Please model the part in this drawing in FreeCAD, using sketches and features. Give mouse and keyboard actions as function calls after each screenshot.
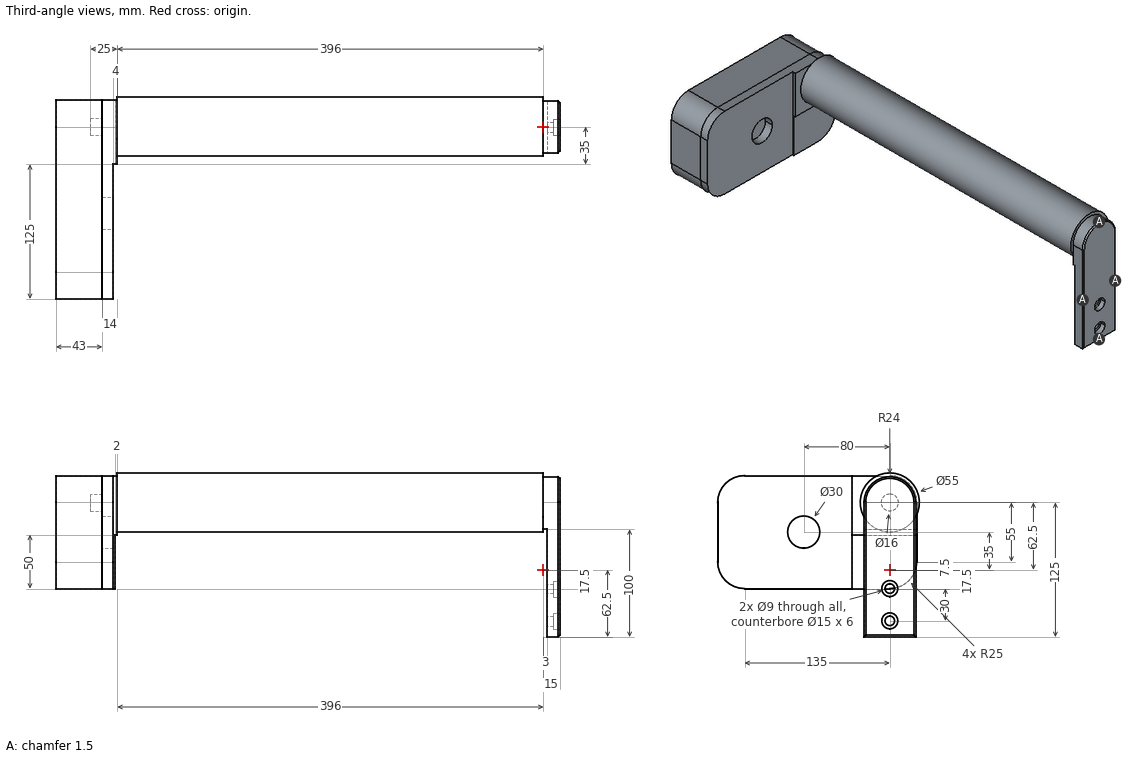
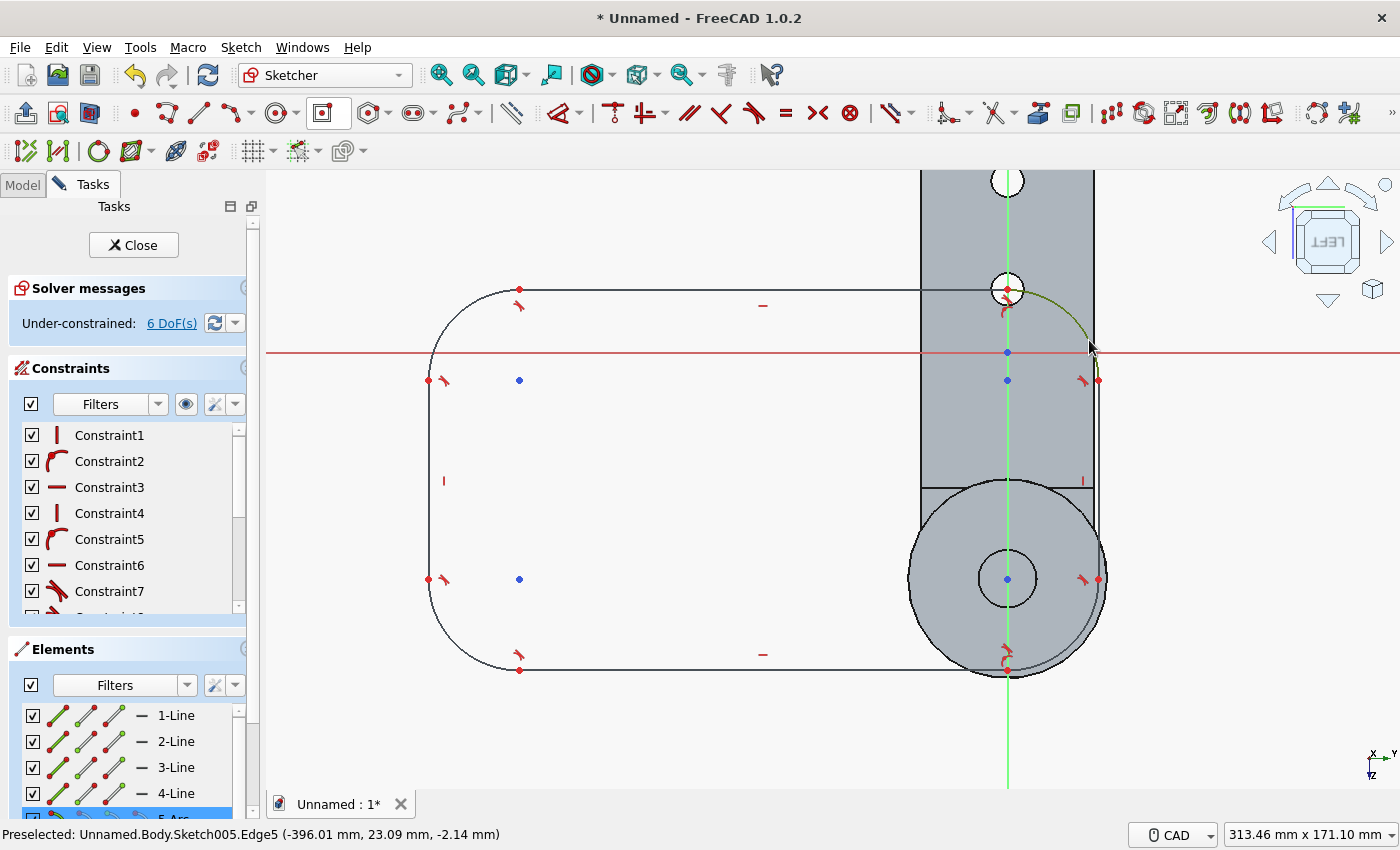
click(479, 300)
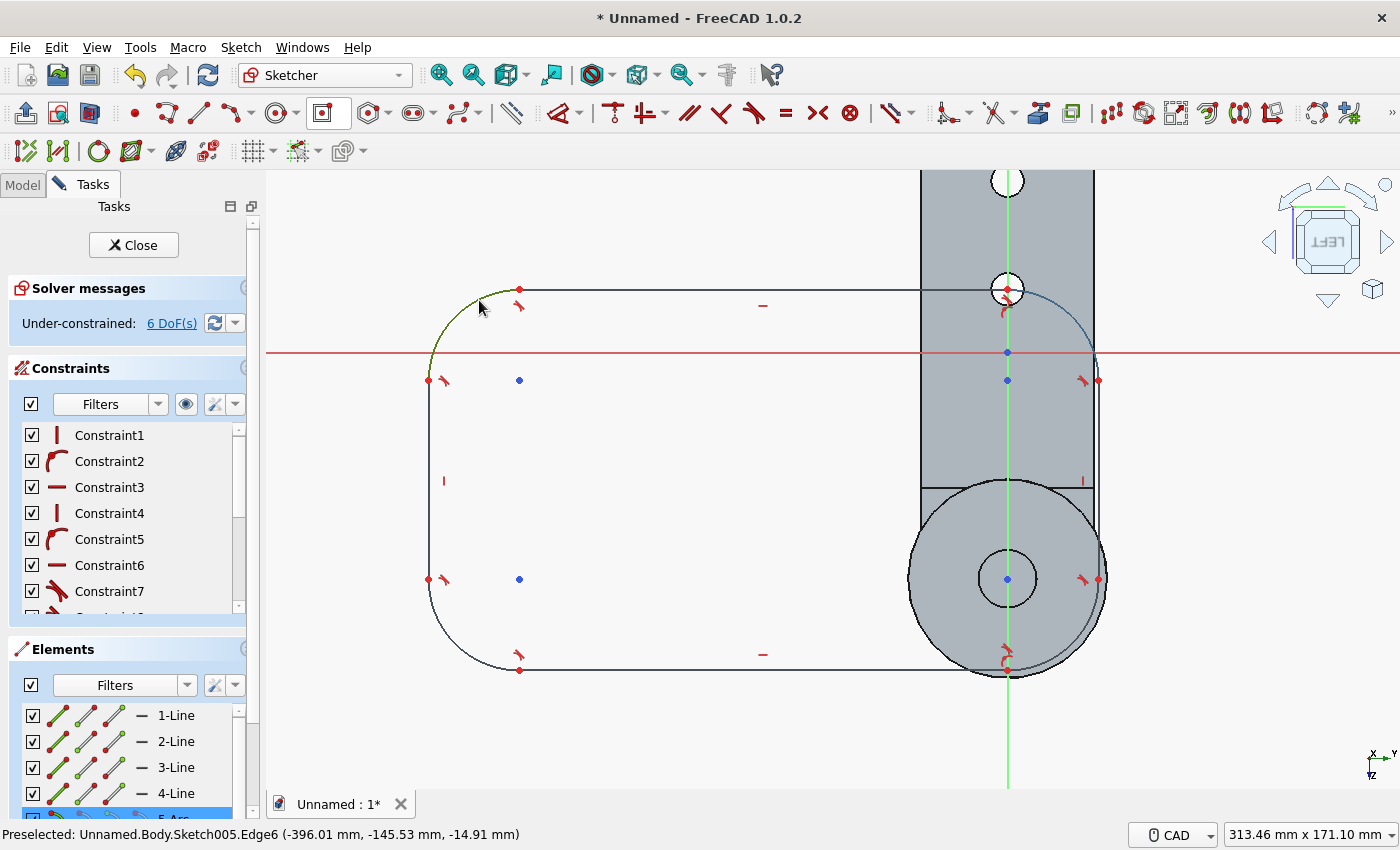
click(439, 621)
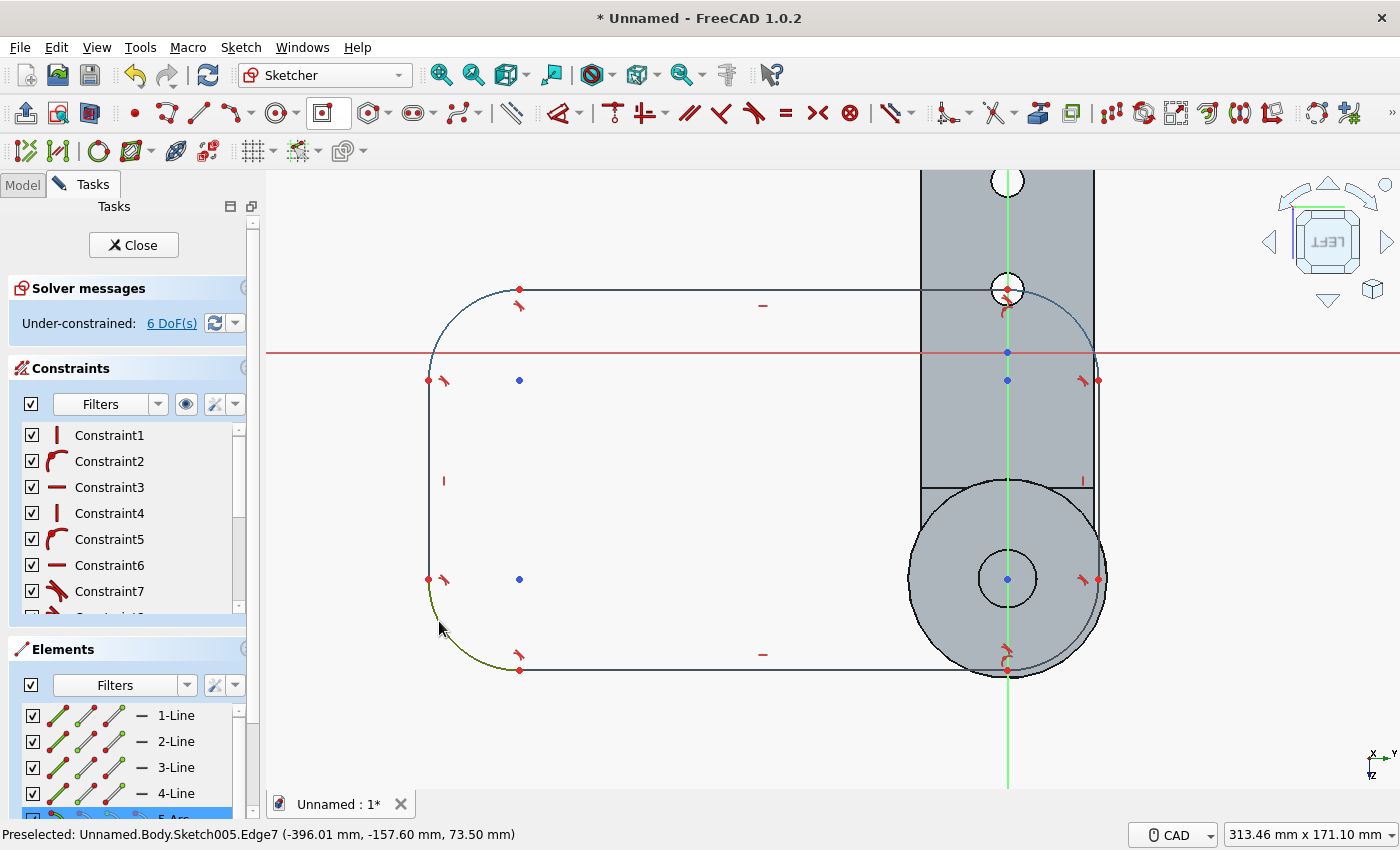
key(e)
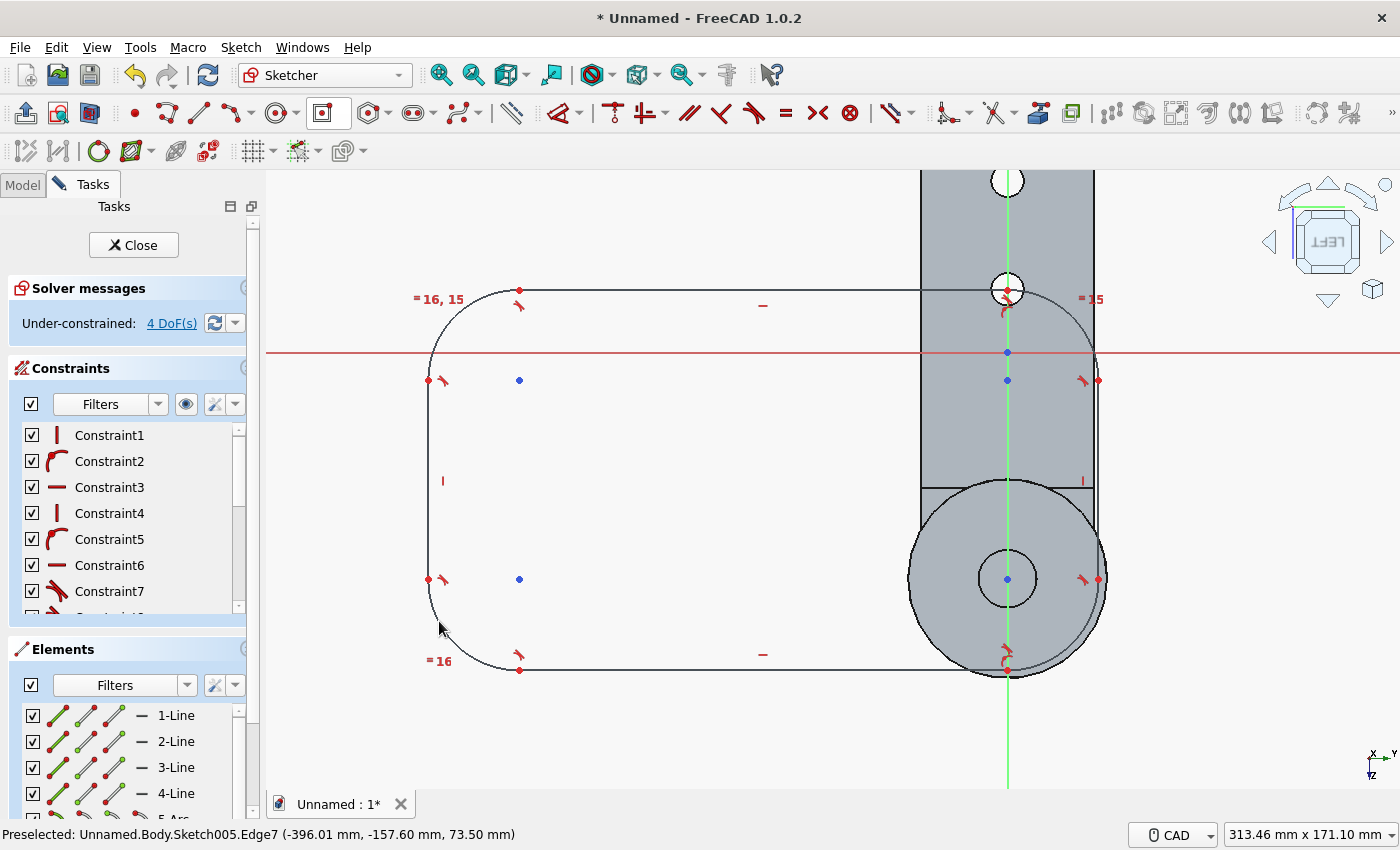
click(558, 114)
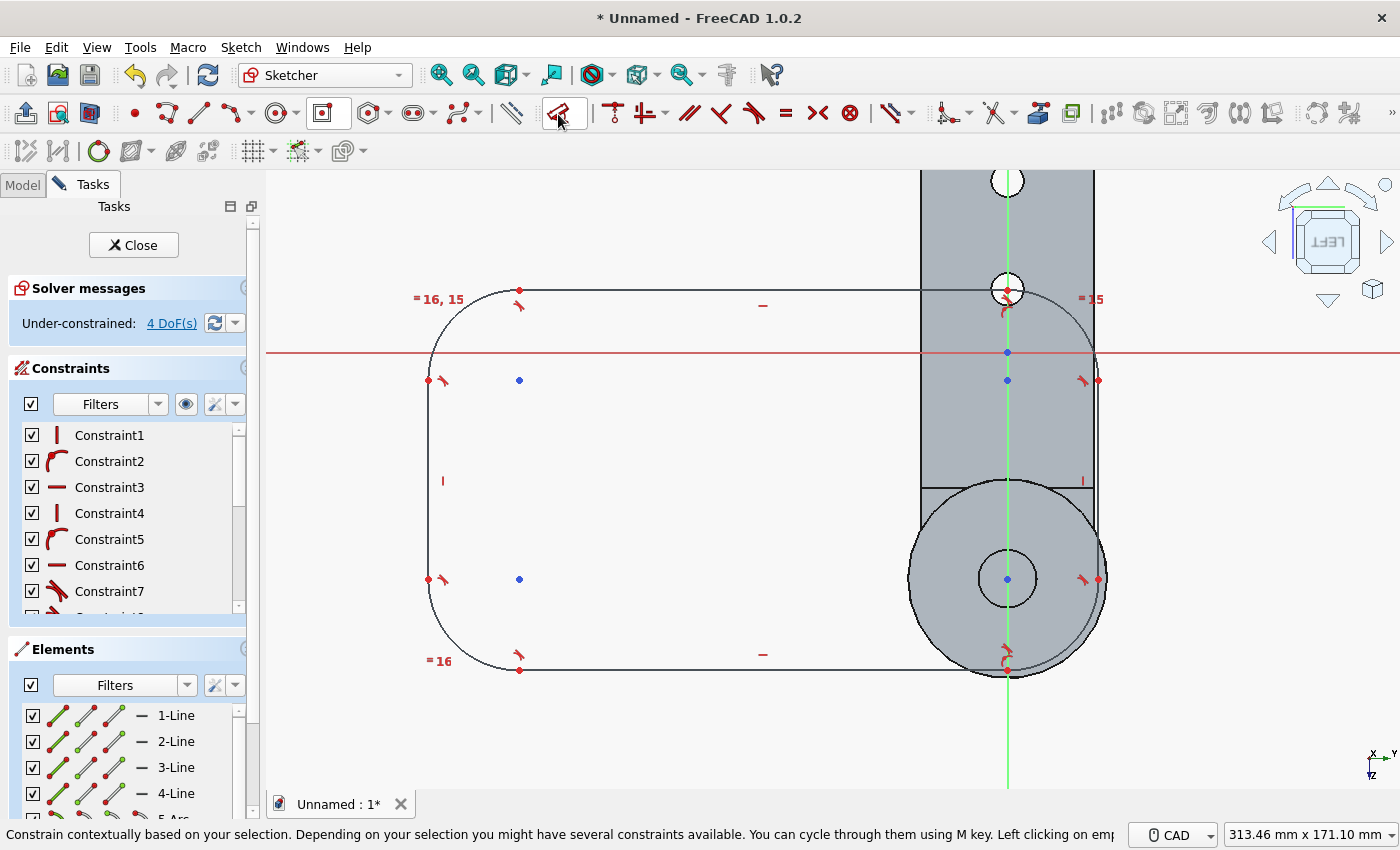
click(1089, 340)
click(1118, 326)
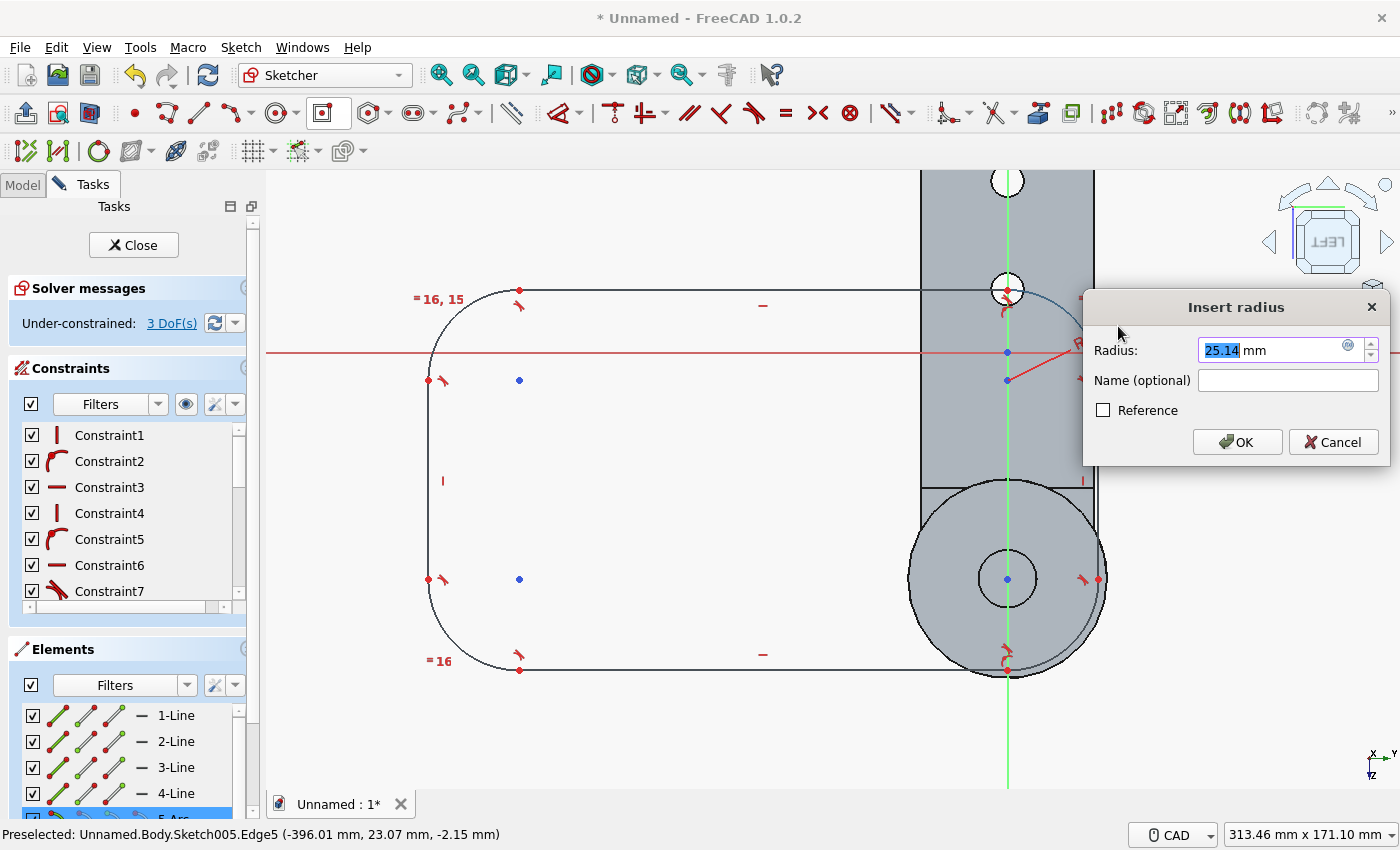
text(25)
key(Return)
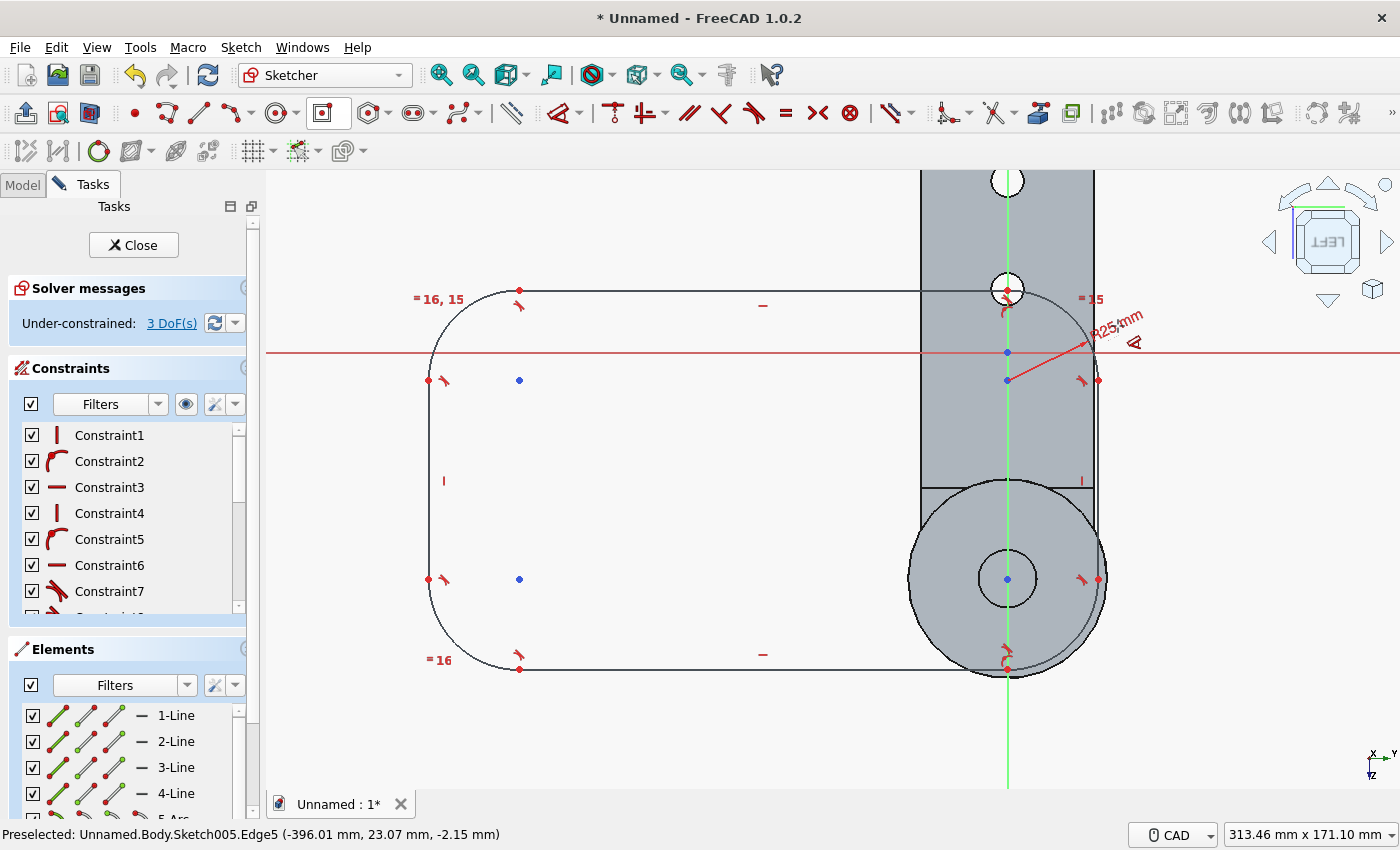
click(1098, 520)
click(1132, 480)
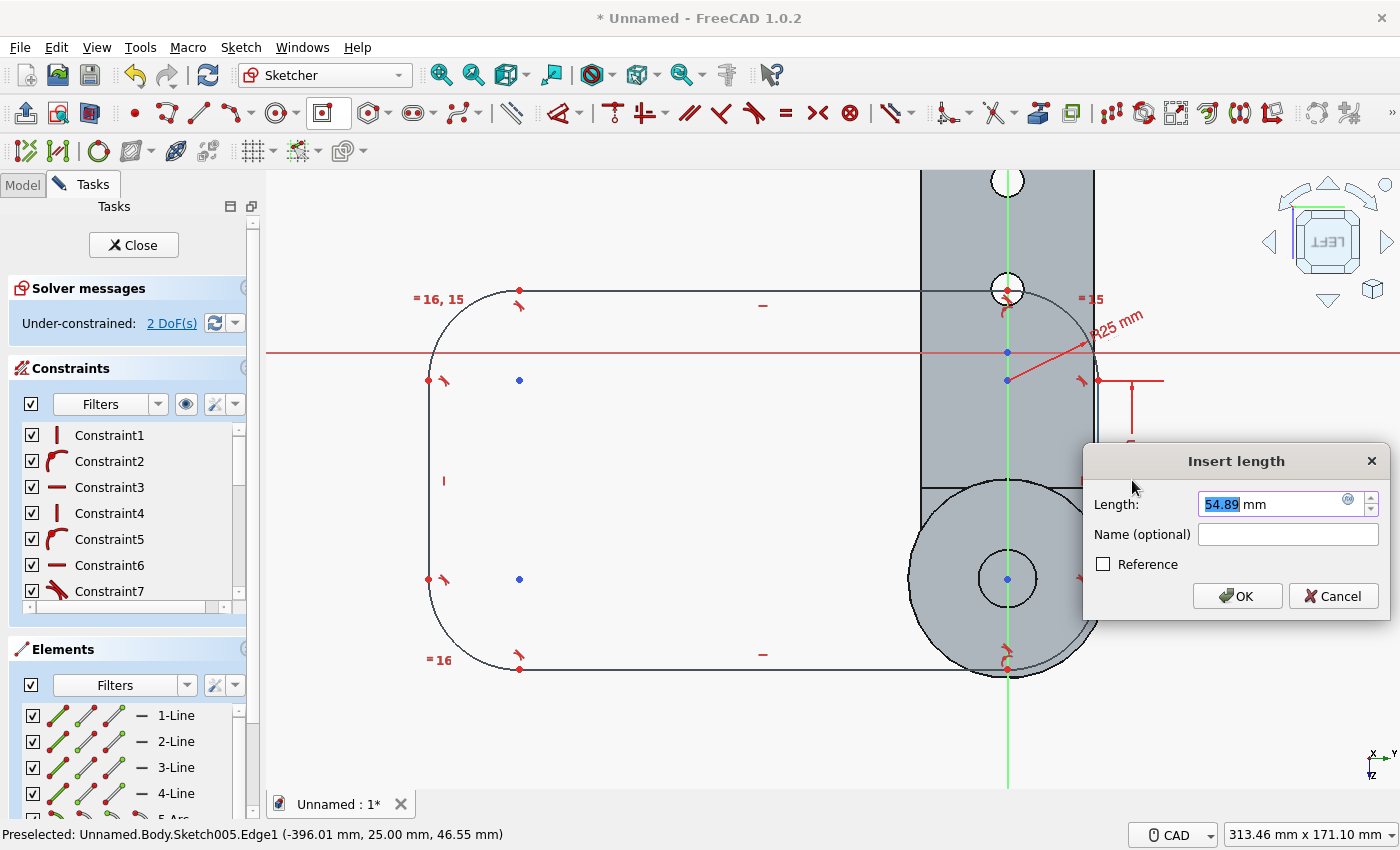
text(55)
key(Return)